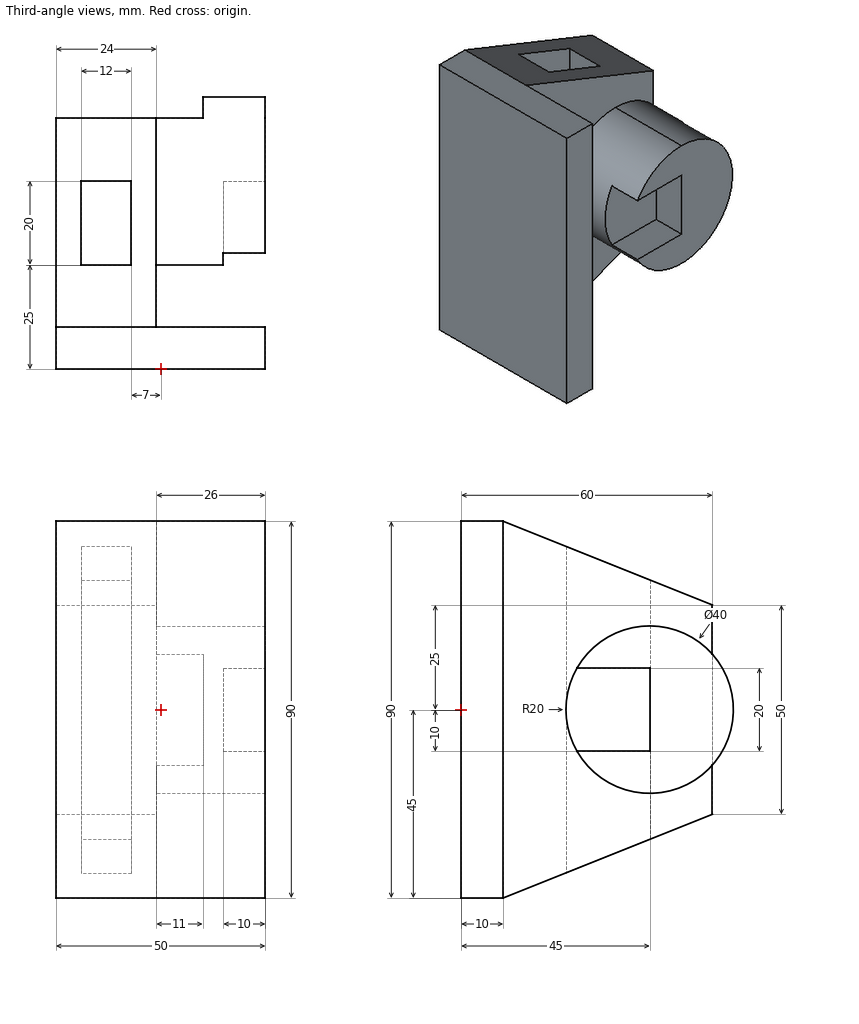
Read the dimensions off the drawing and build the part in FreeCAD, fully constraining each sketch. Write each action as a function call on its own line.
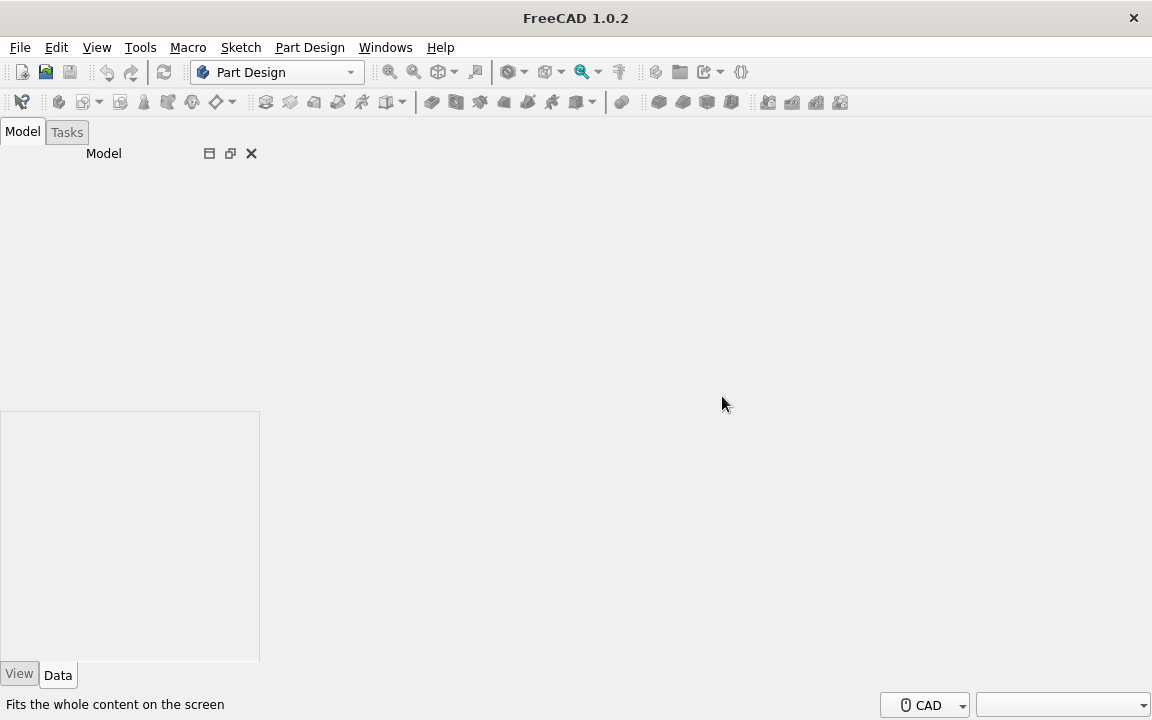
click(22, 72)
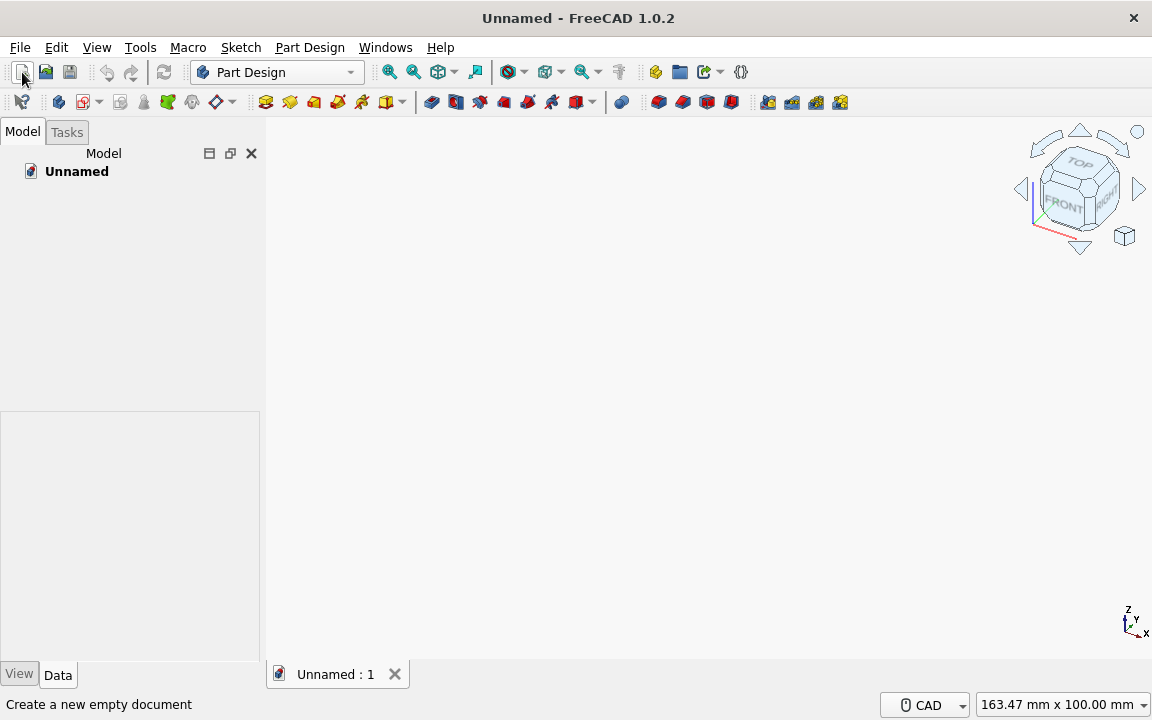
click(84, 102)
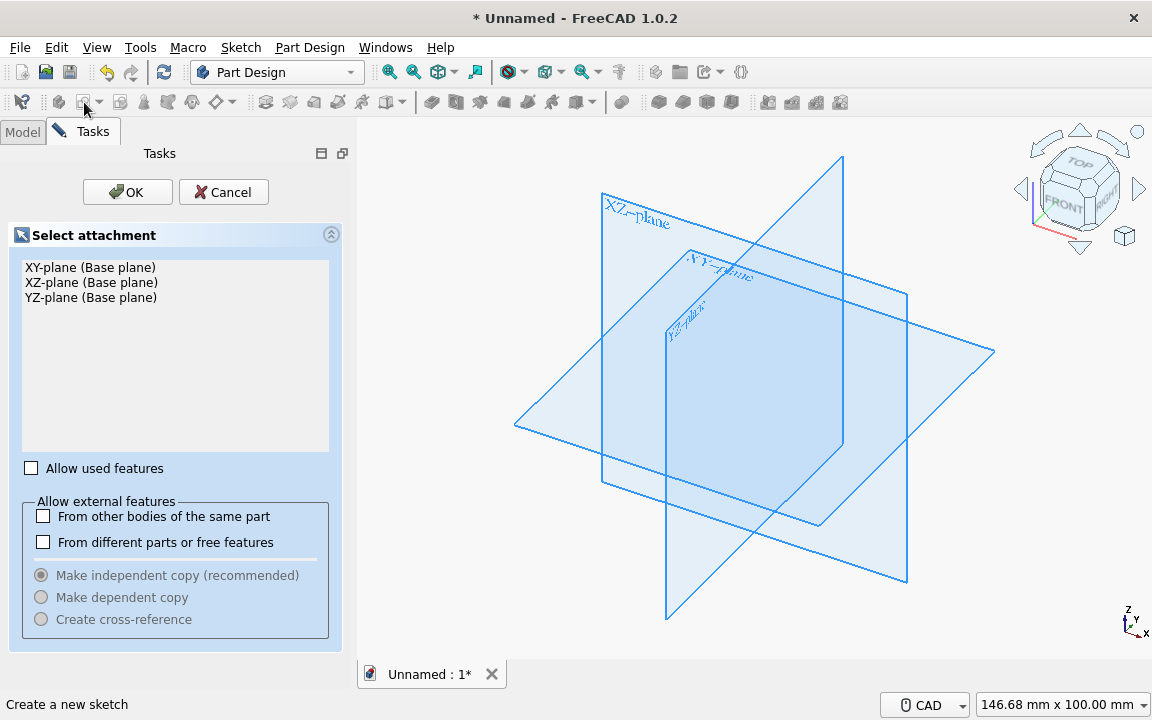
click(82, 282)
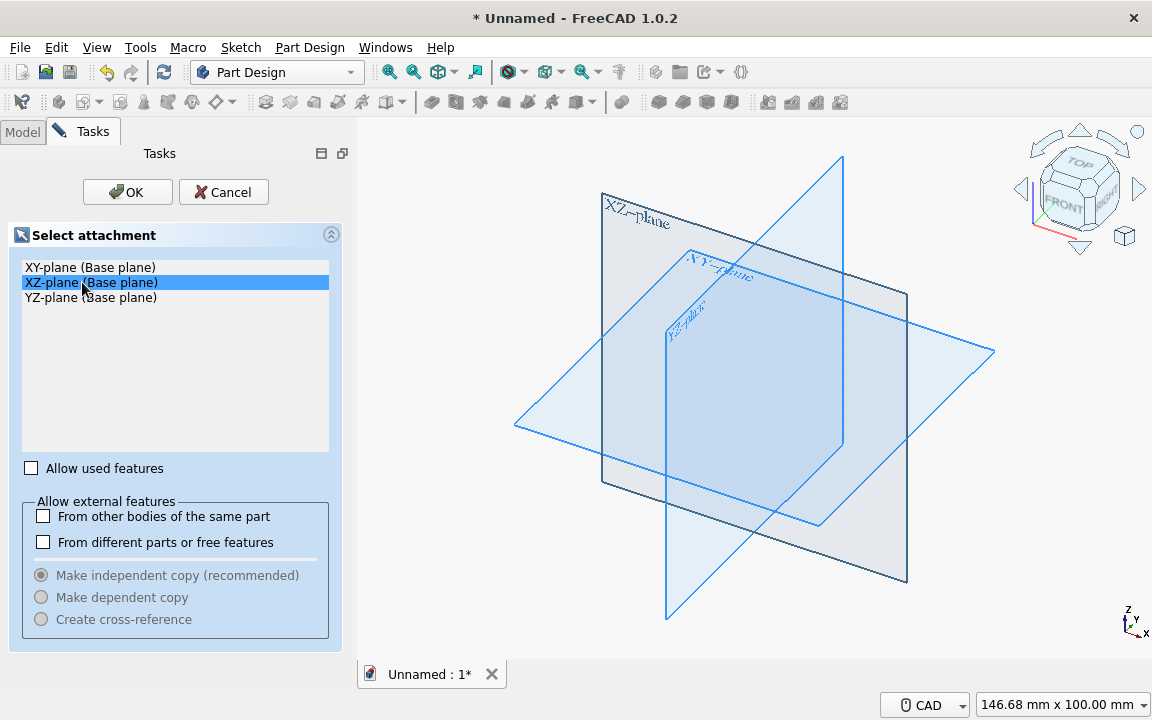
click(128, 192)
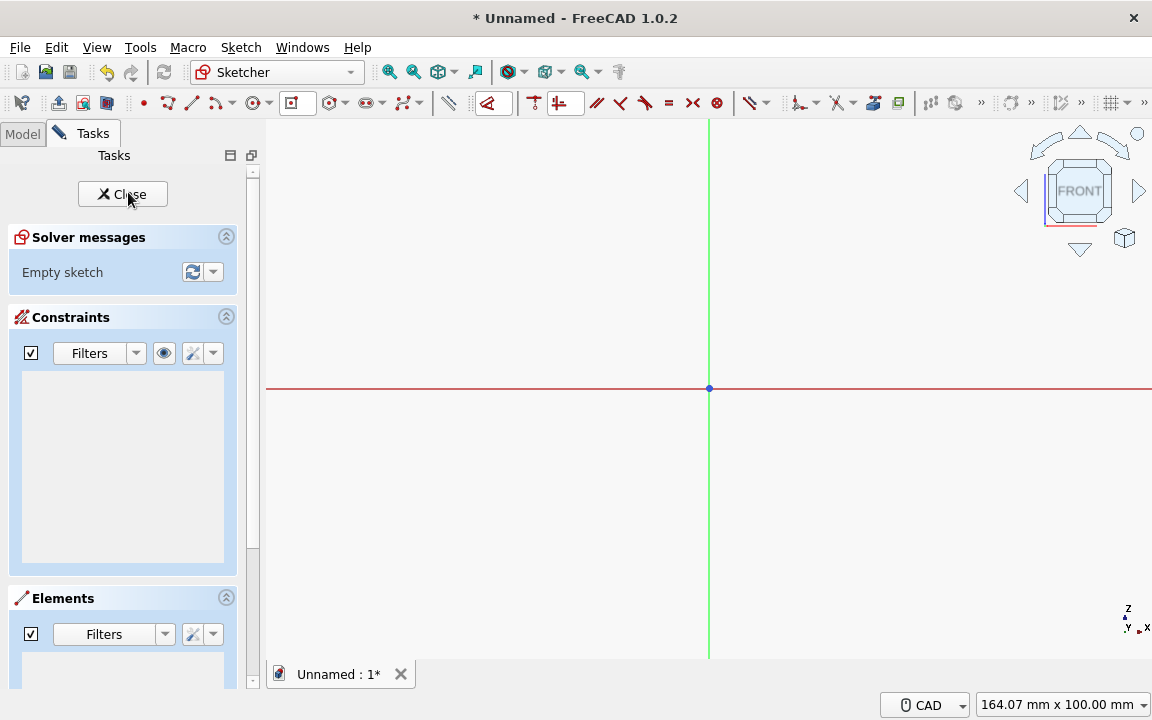
scroll(501, 389, down, 2)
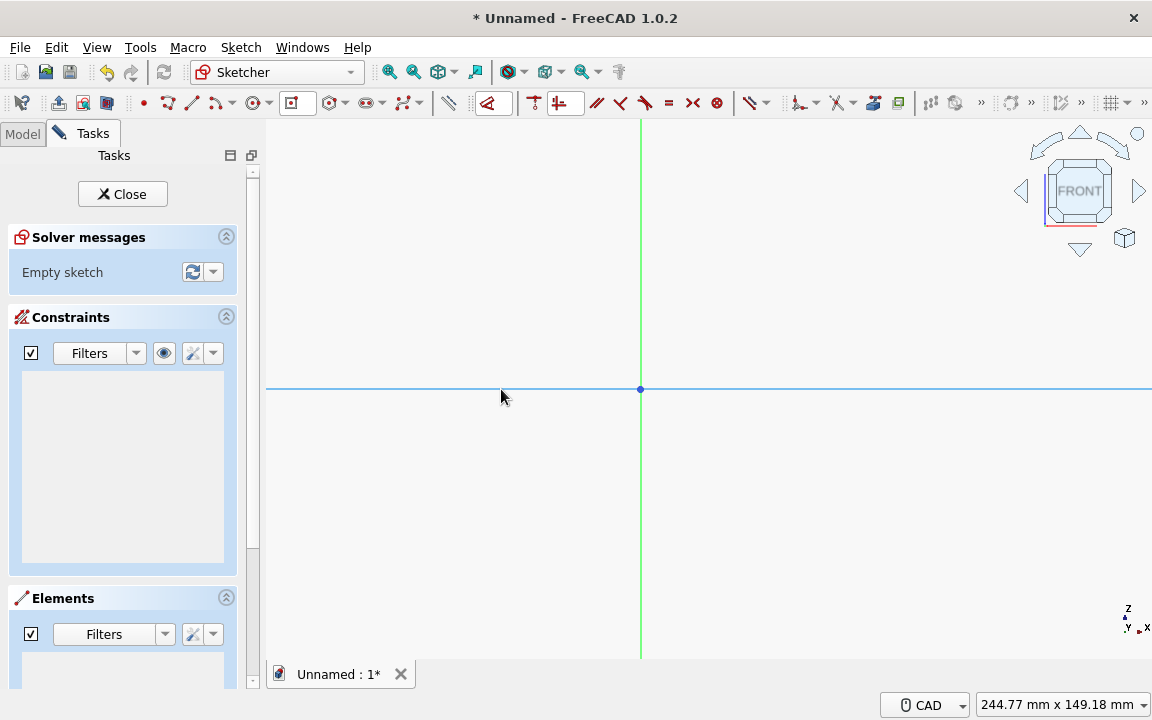
key(g)
key(v)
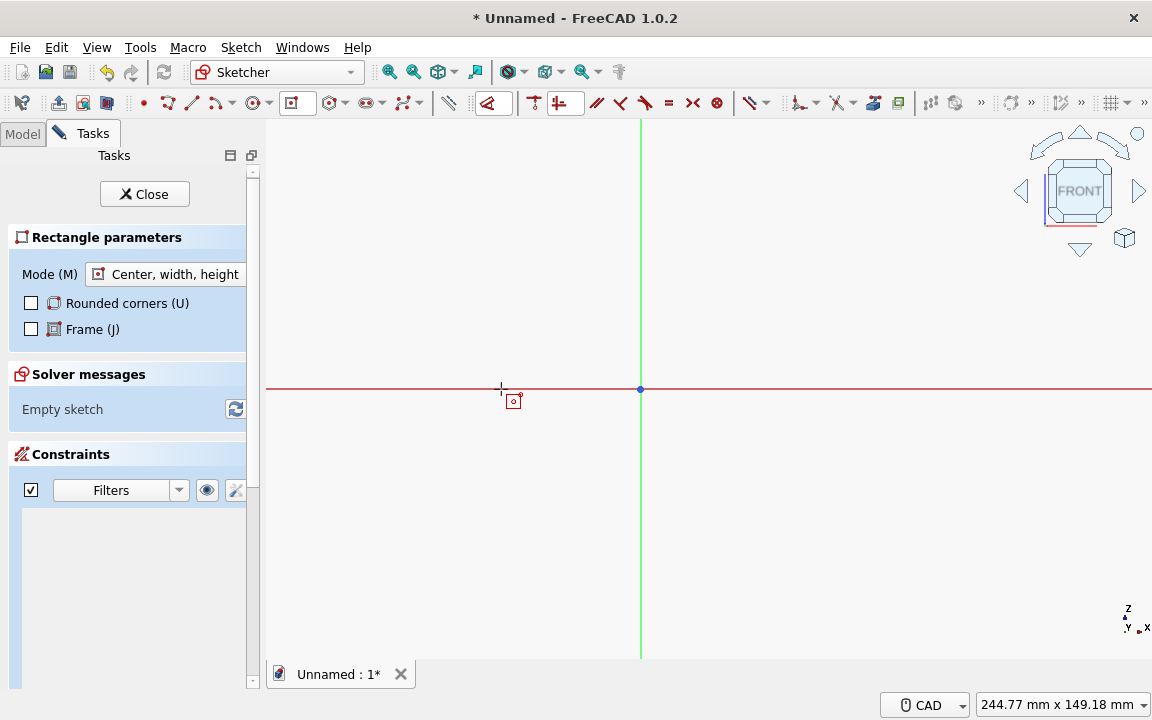
click(641, 389)
move(731, 226)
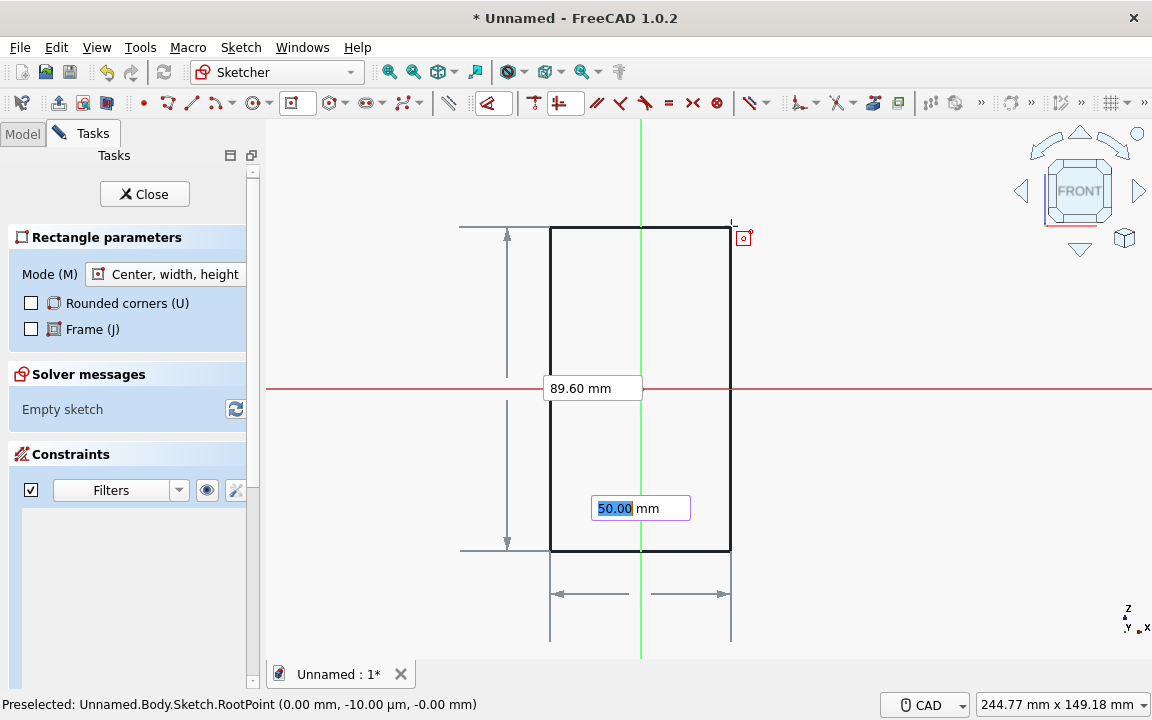
text(50)
key(Tab)
text(90)
key(Return)
key(Escape)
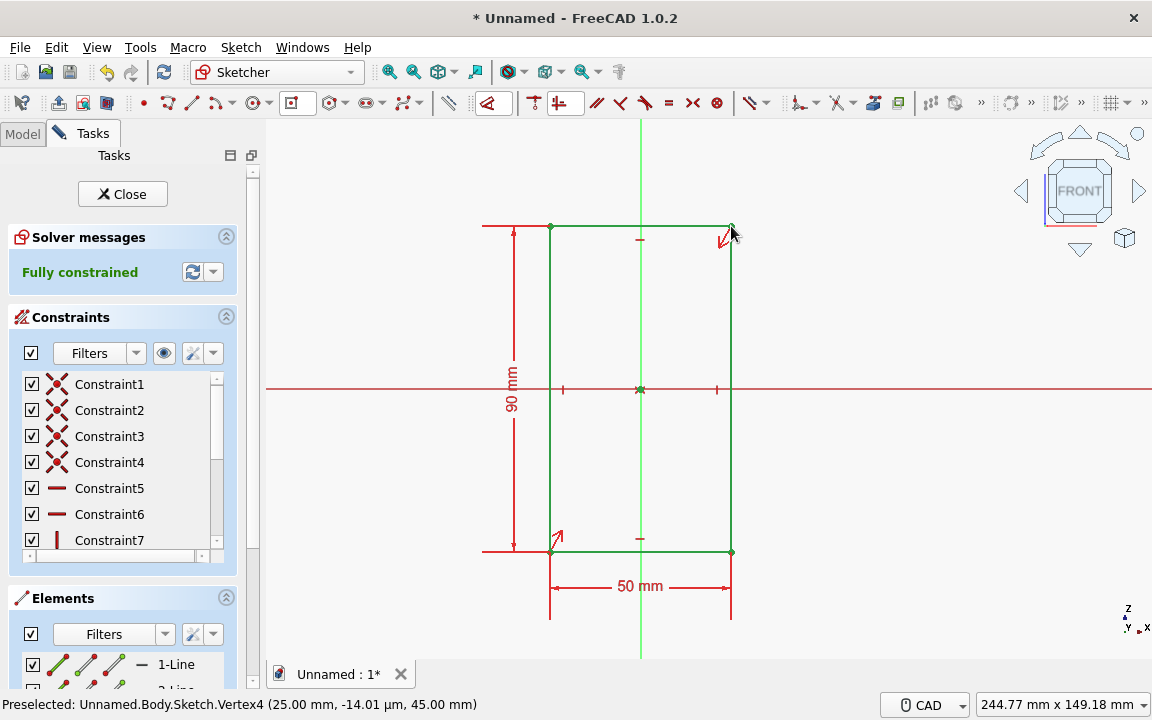
click(123, 194)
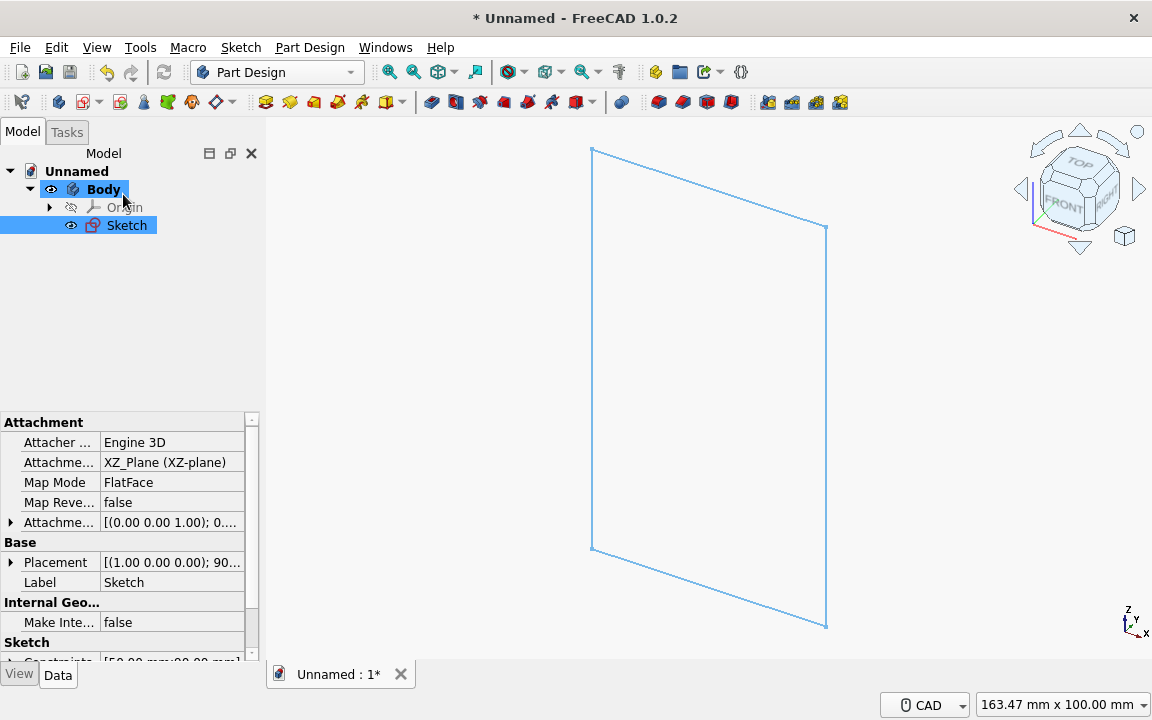
click(266, 102)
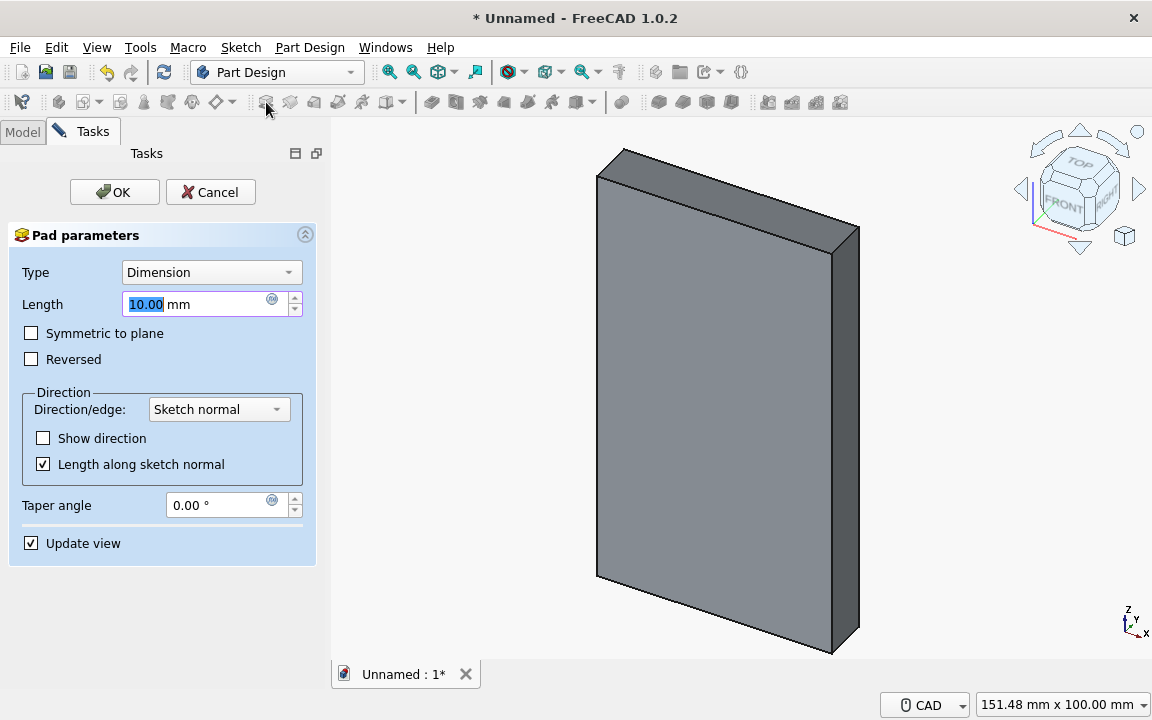
text(10)
key(Tab)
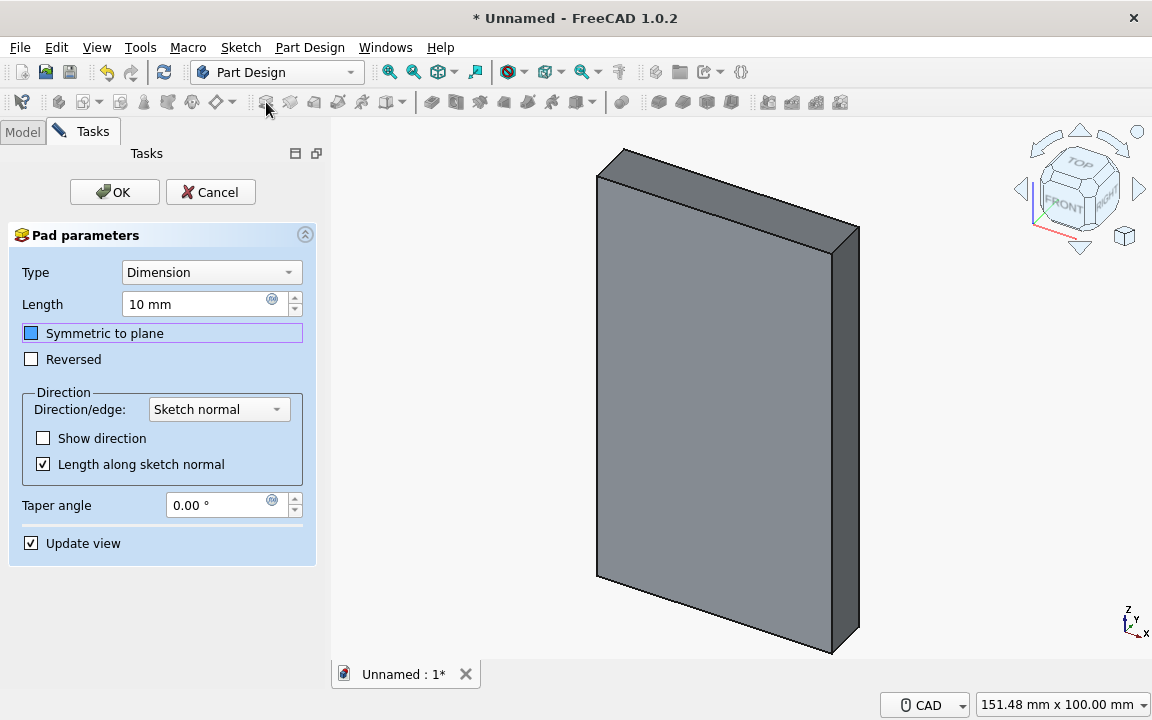
click(30, 359)